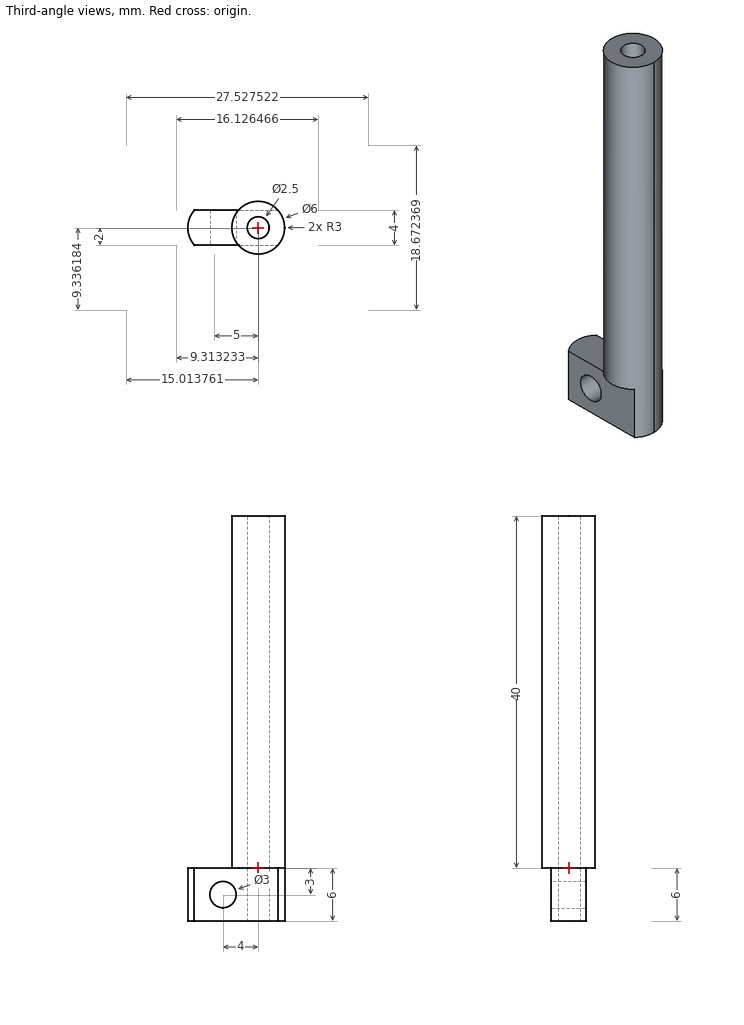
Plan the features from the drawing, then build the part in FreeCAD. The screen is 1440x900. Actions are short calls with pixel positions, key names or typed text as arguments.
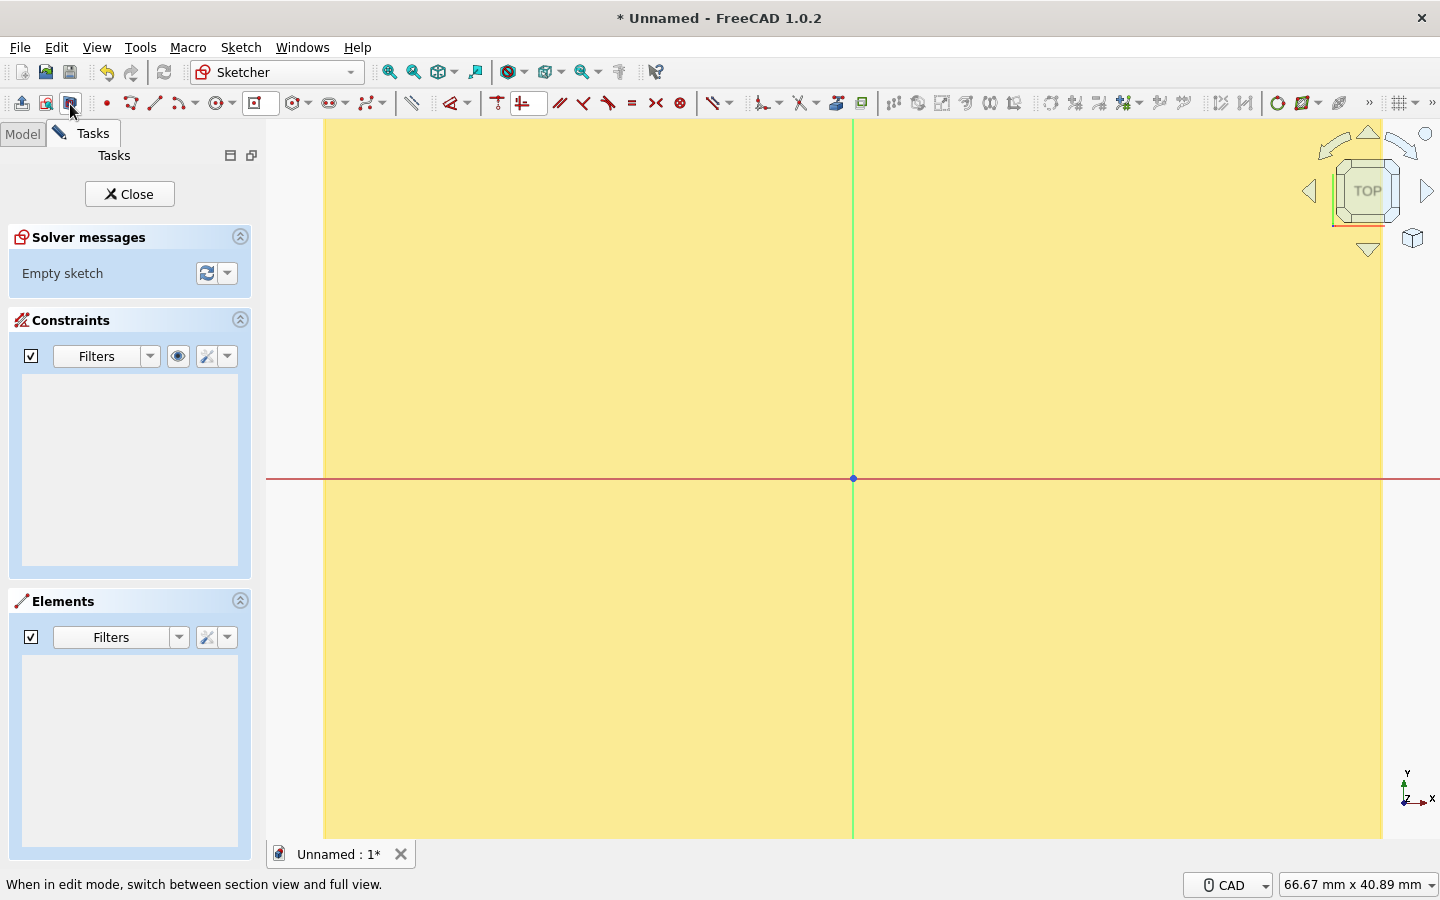
scroll(820, 479, up, 6)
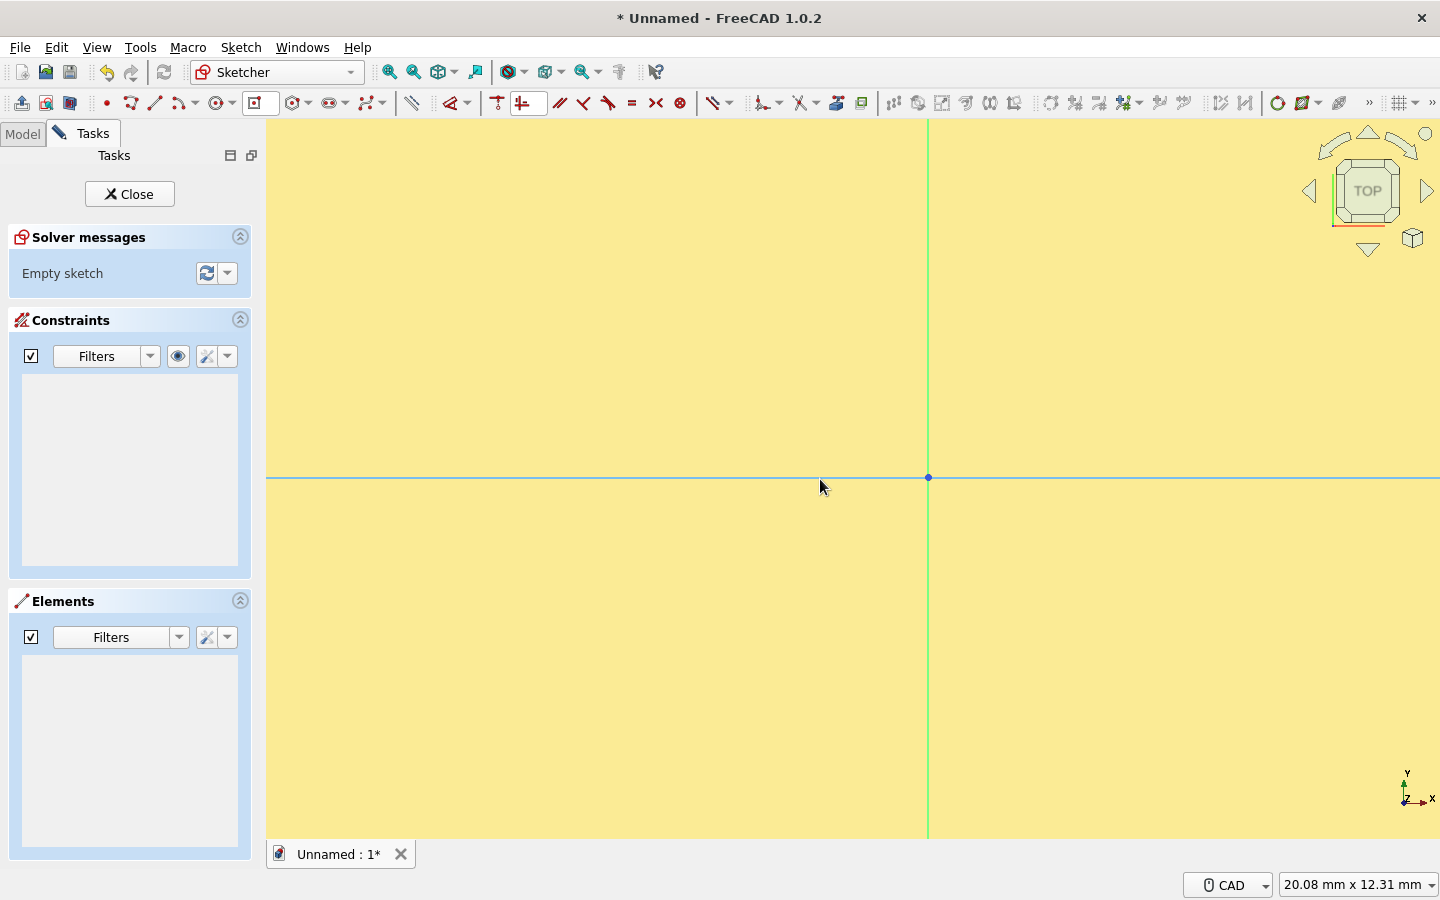
key(g)
key(s)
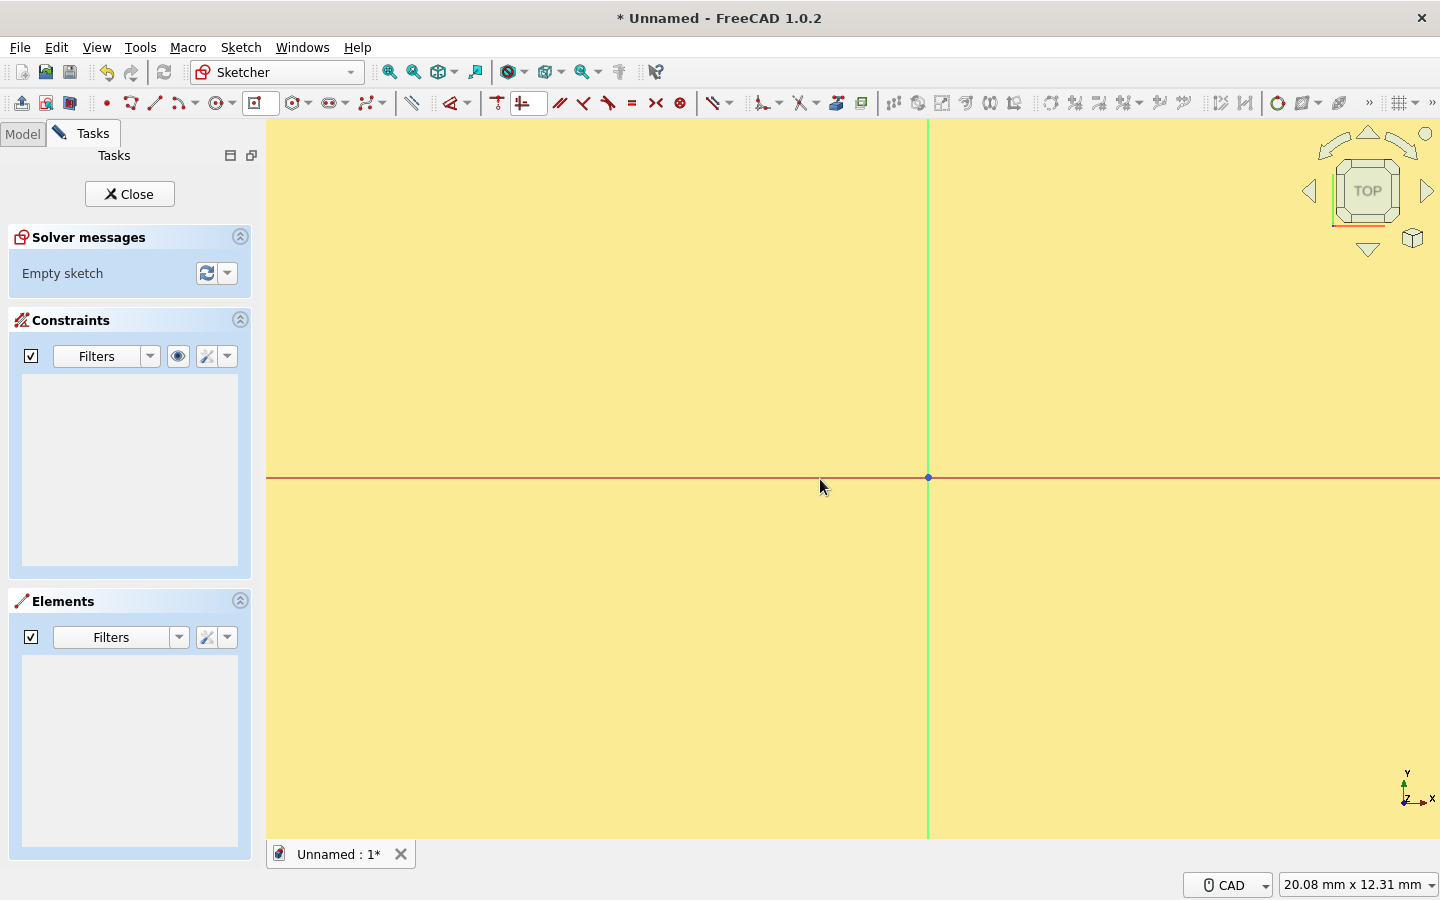
click(928, 478)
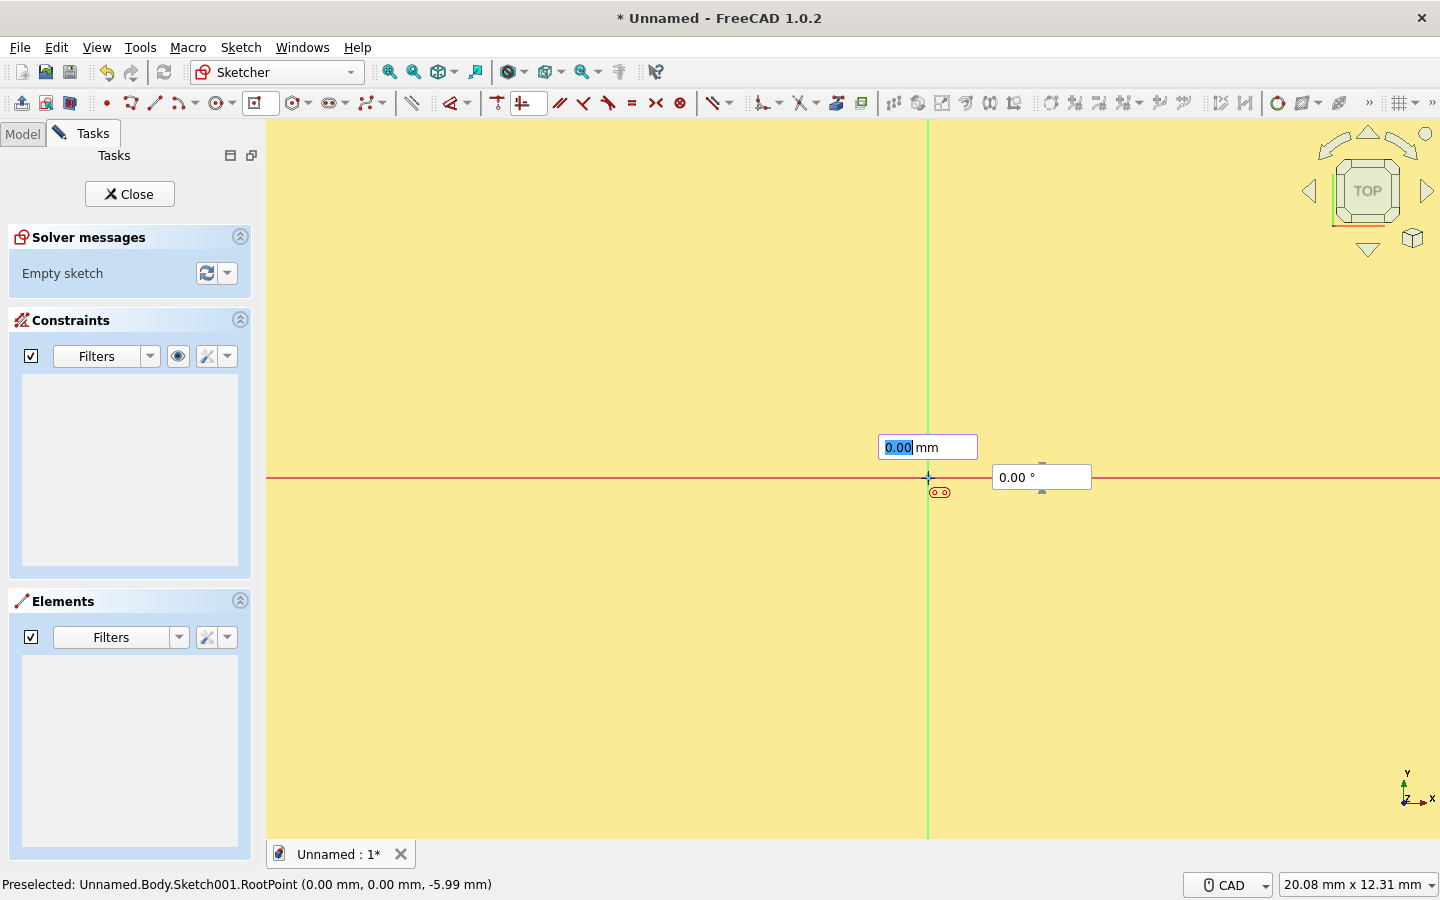
click(636, 469)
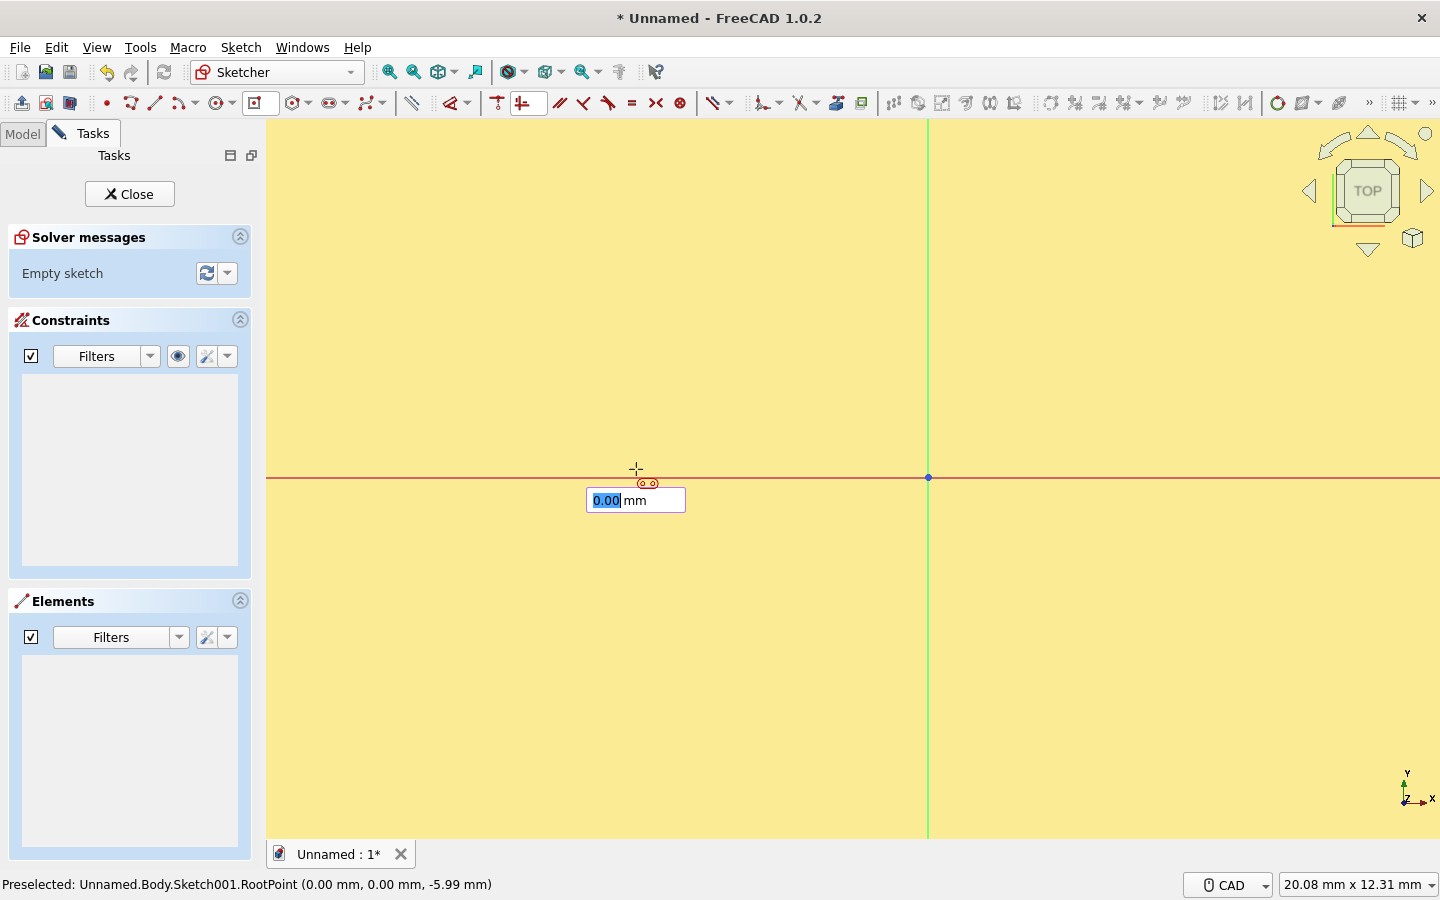
click(782, 302)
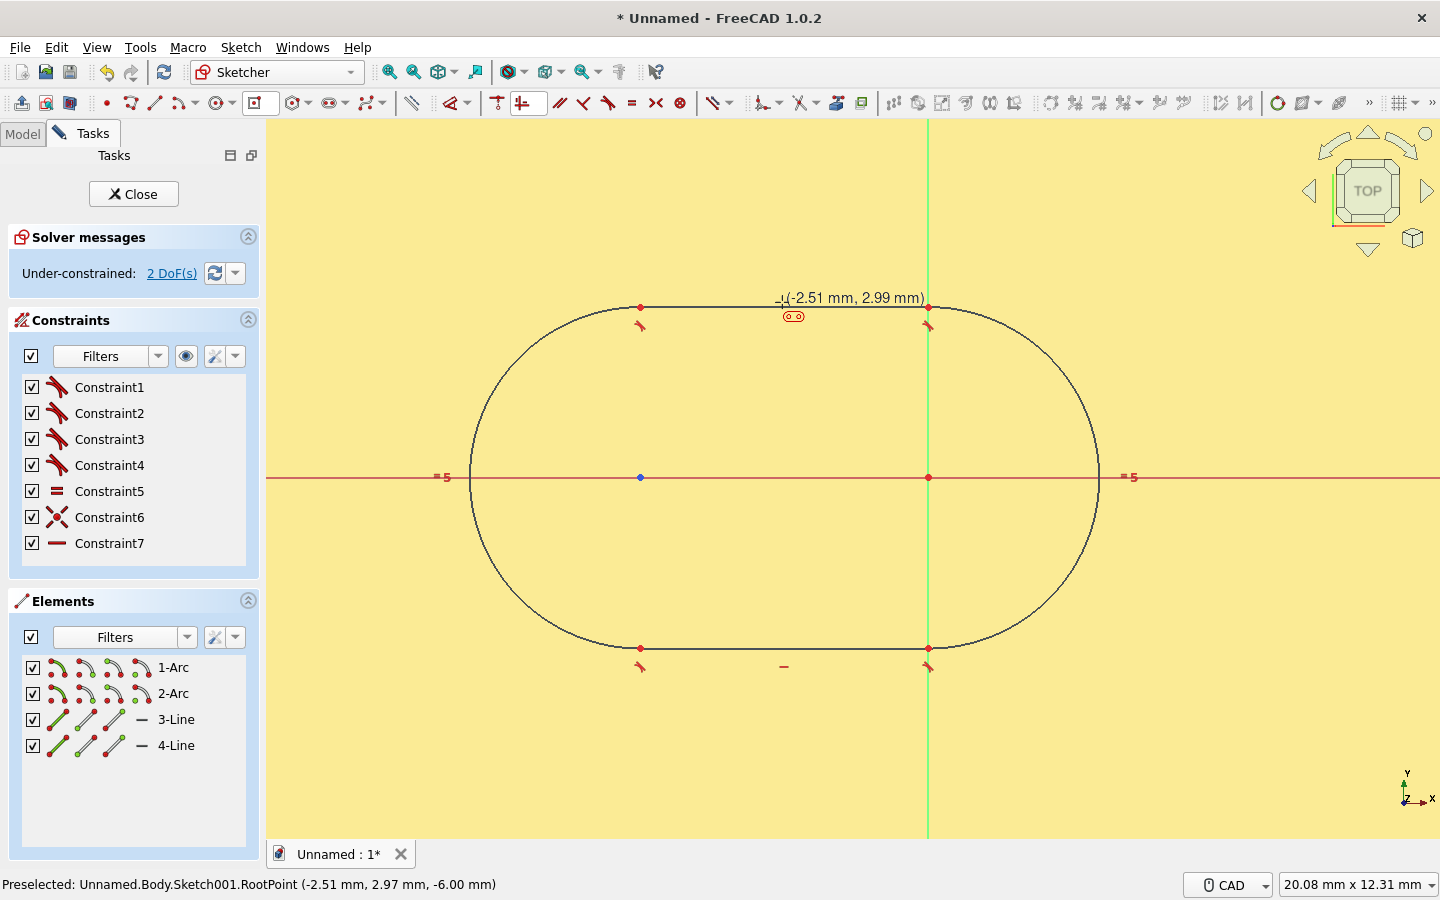
key(g)
key(c)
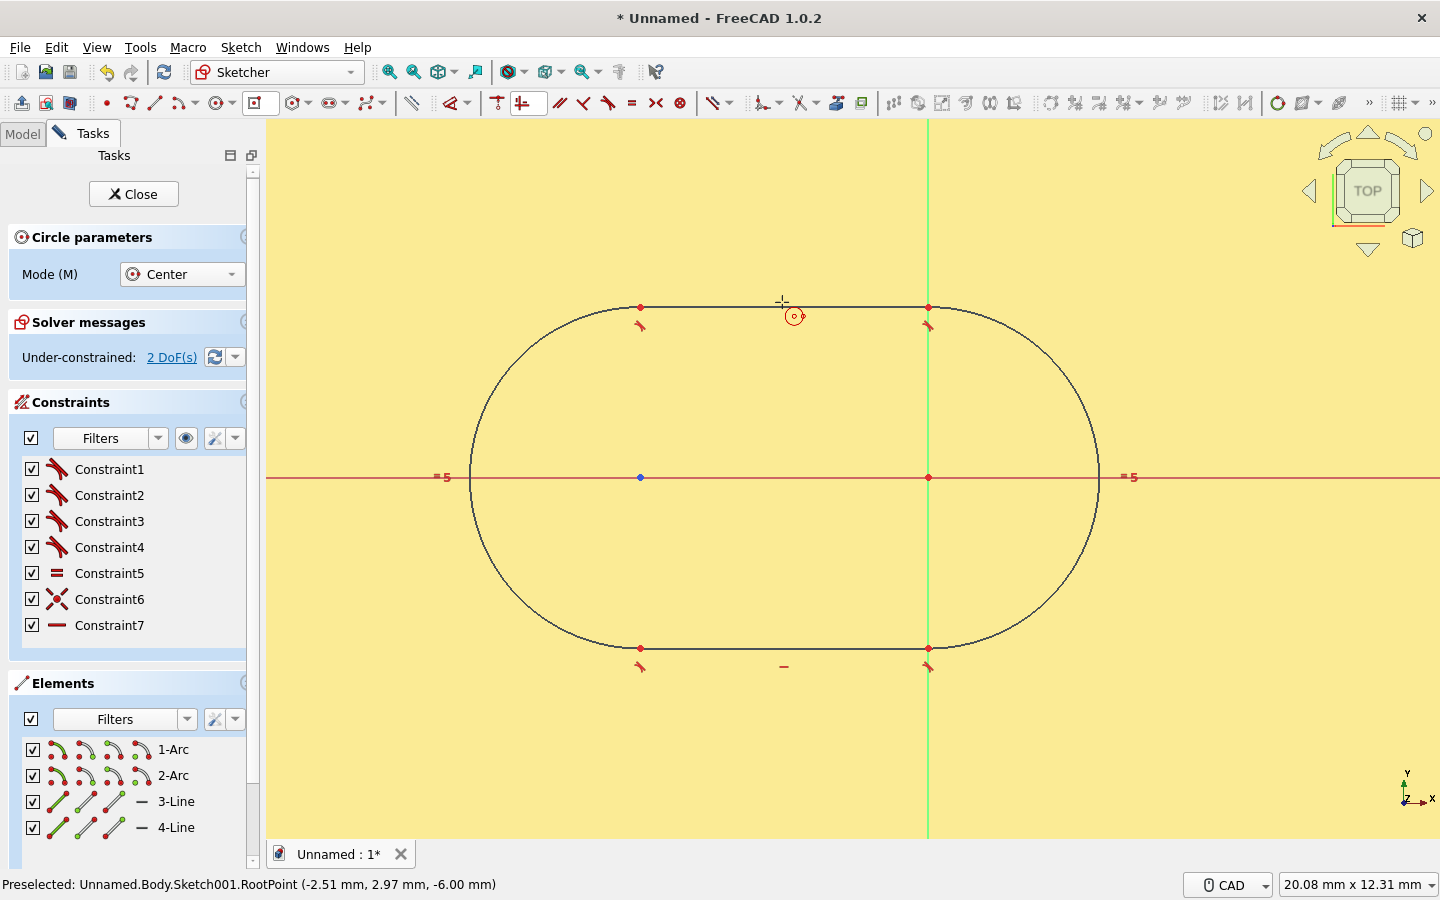
click(928, 478)
move(980, 426)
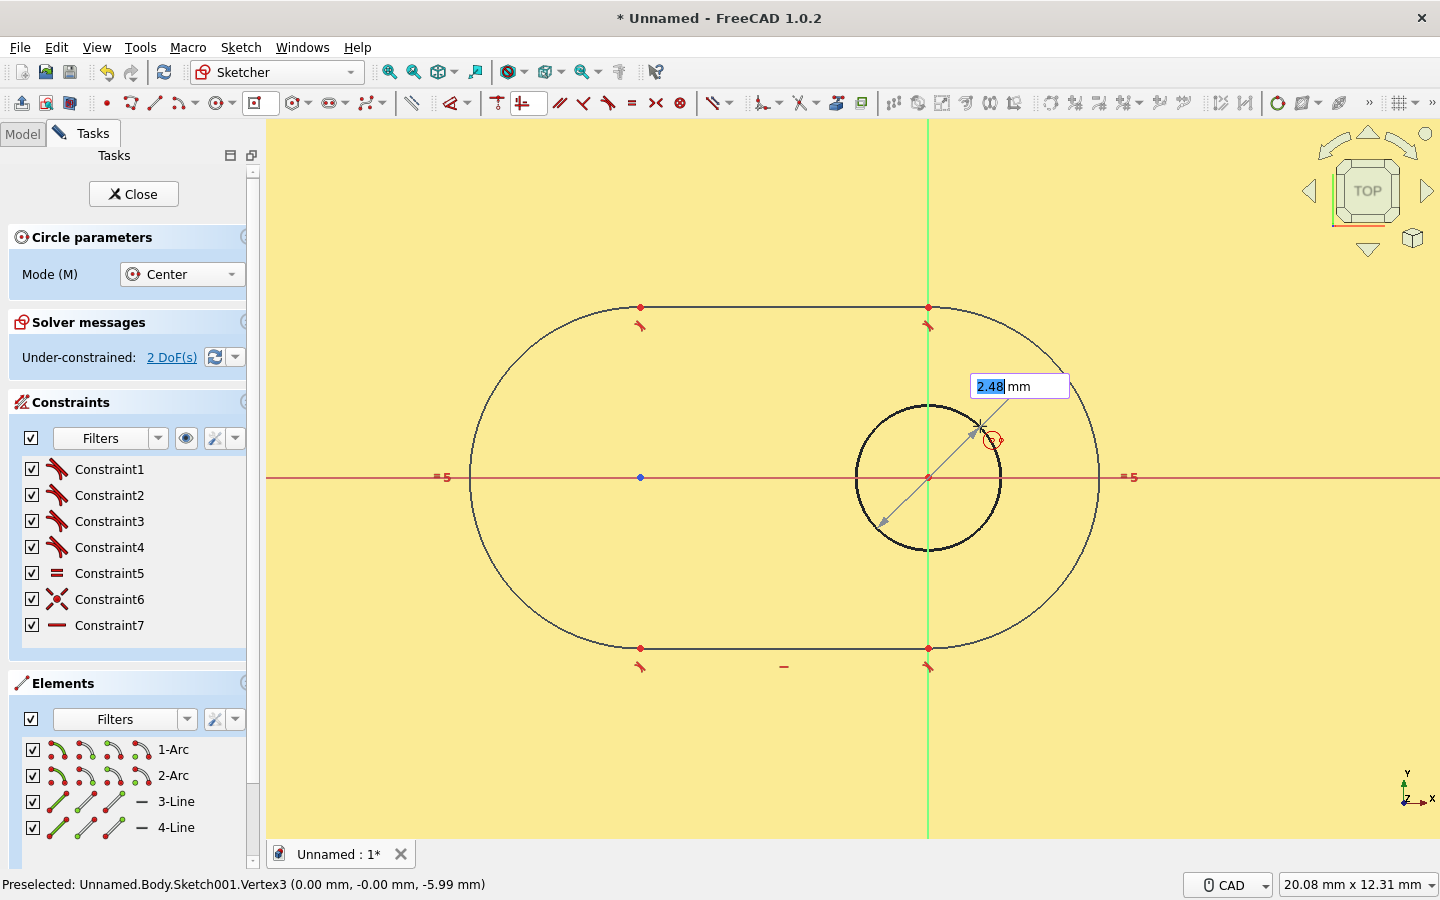
text(2.5)
key(Return)
key(Escape)